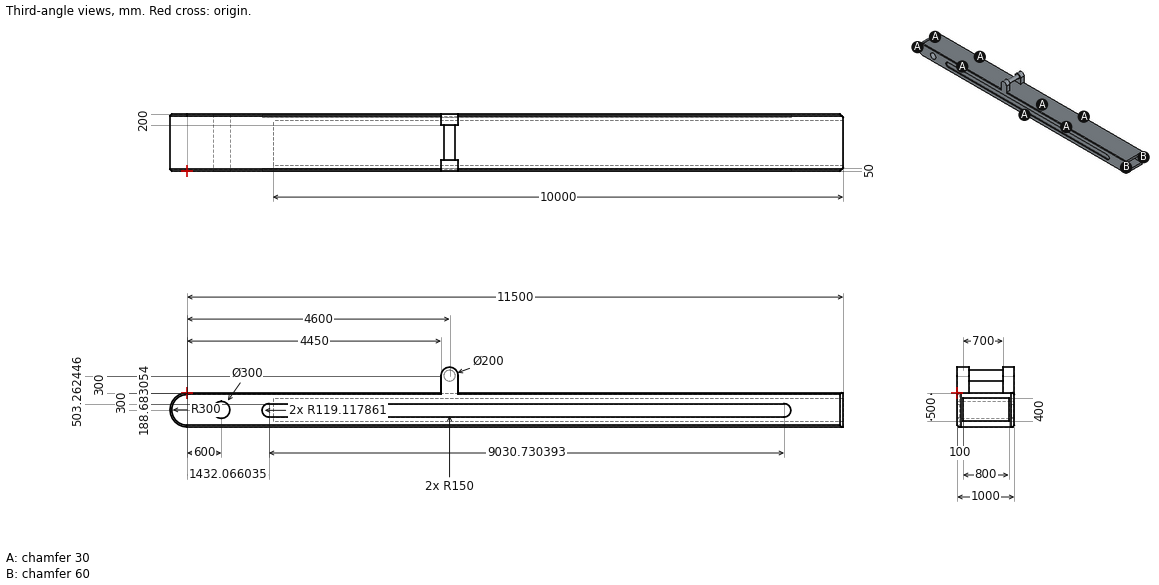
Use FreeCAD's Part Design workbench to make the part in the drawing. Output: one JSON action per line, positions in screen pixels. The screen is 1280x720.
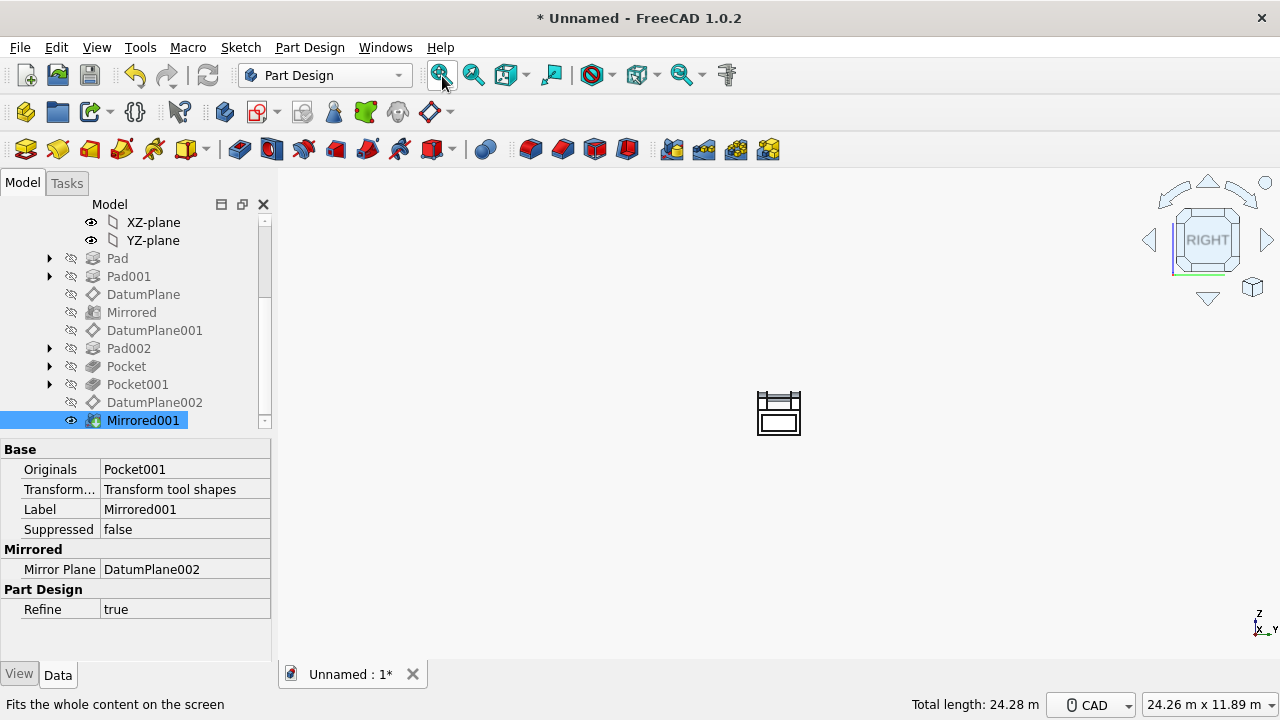
{"action": "key", "text": "5"}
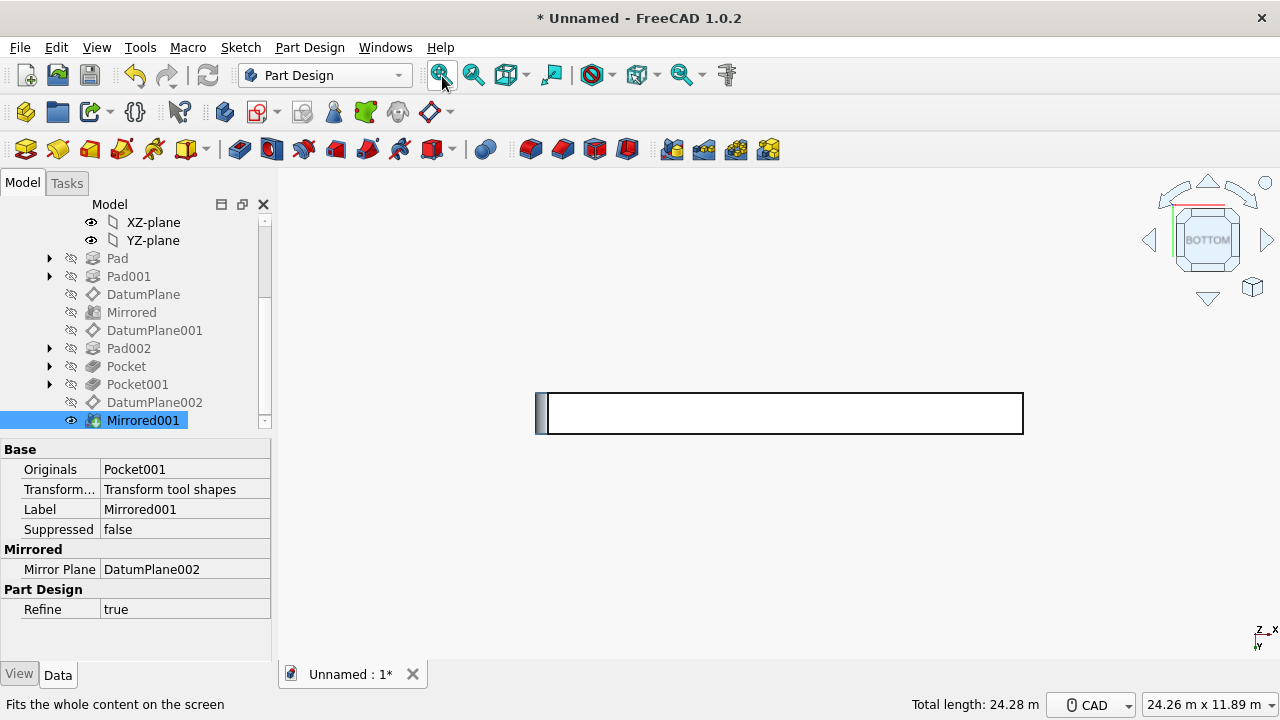
{"action": "left_click", "coordinate": [785, 392], "text": "ctrl"}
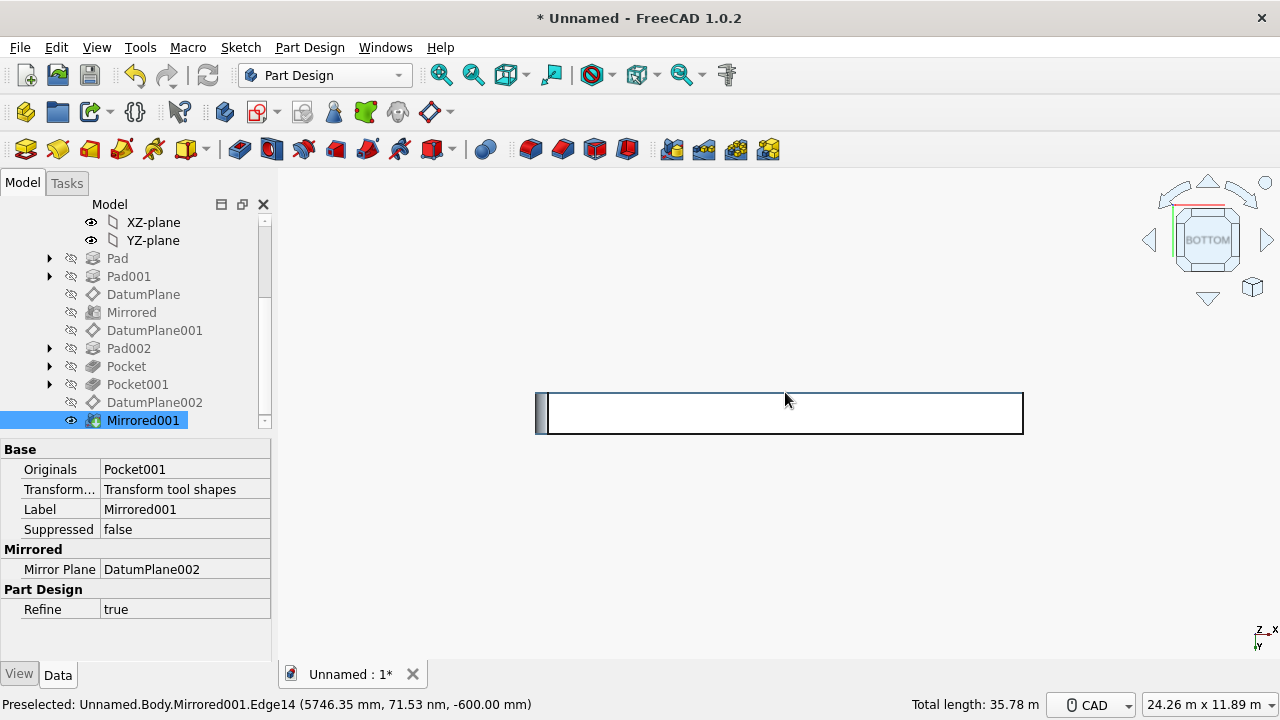
{"action": "key", "text": "4"}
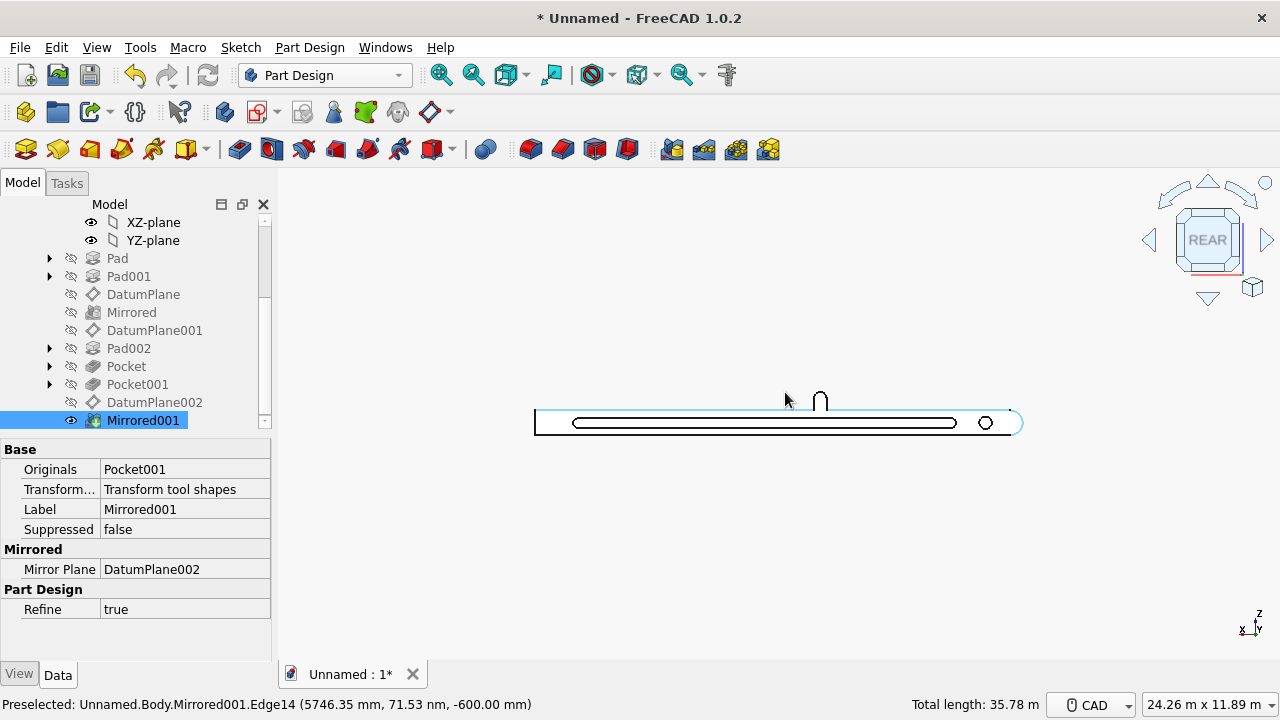
{"action": "left_click", "coordinate": [773, 434], "text": "ctrl"}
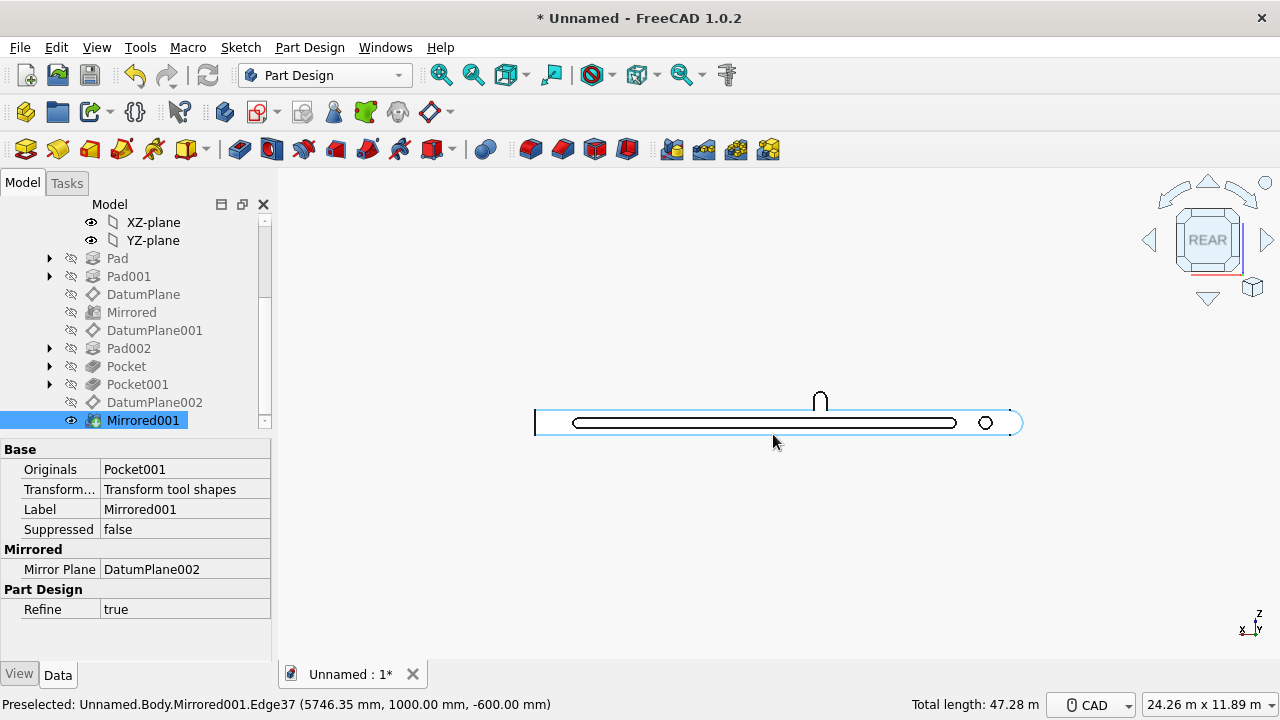
{"action": "left_click", "coordinate": [564, 150]}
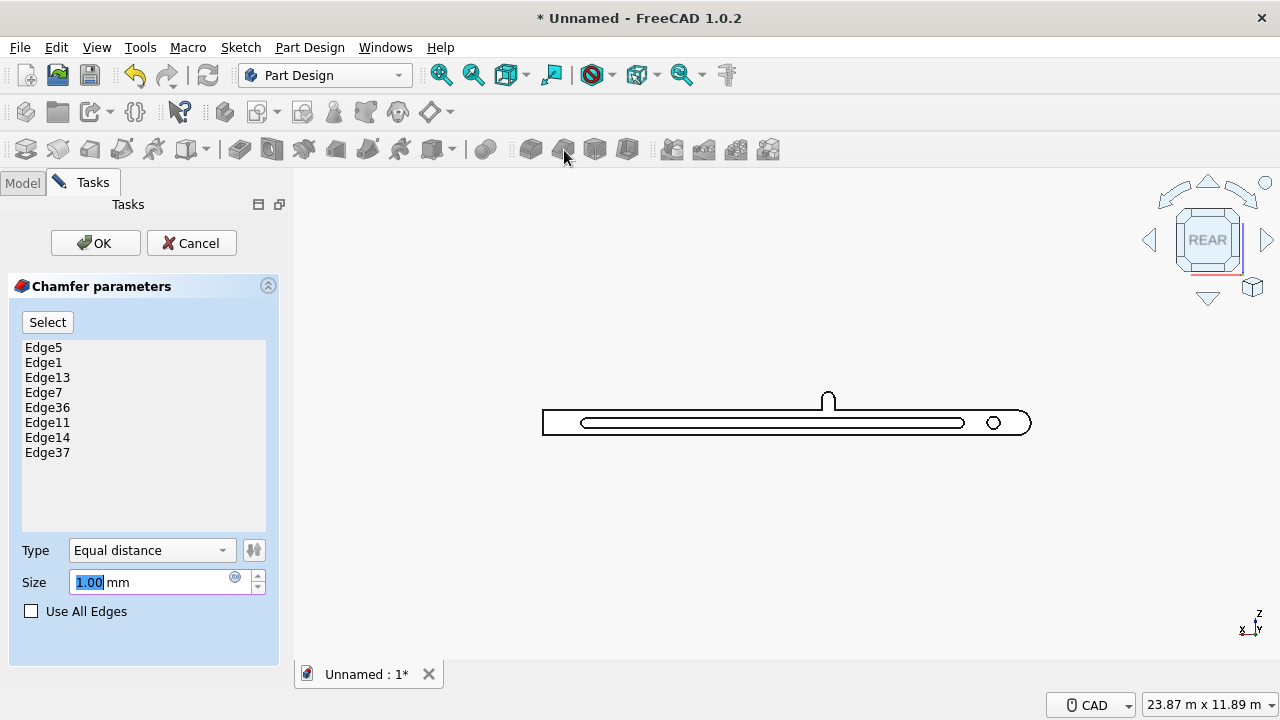
{"action": "type", "text": "30"}
{"action": "key", "text": "Tab"}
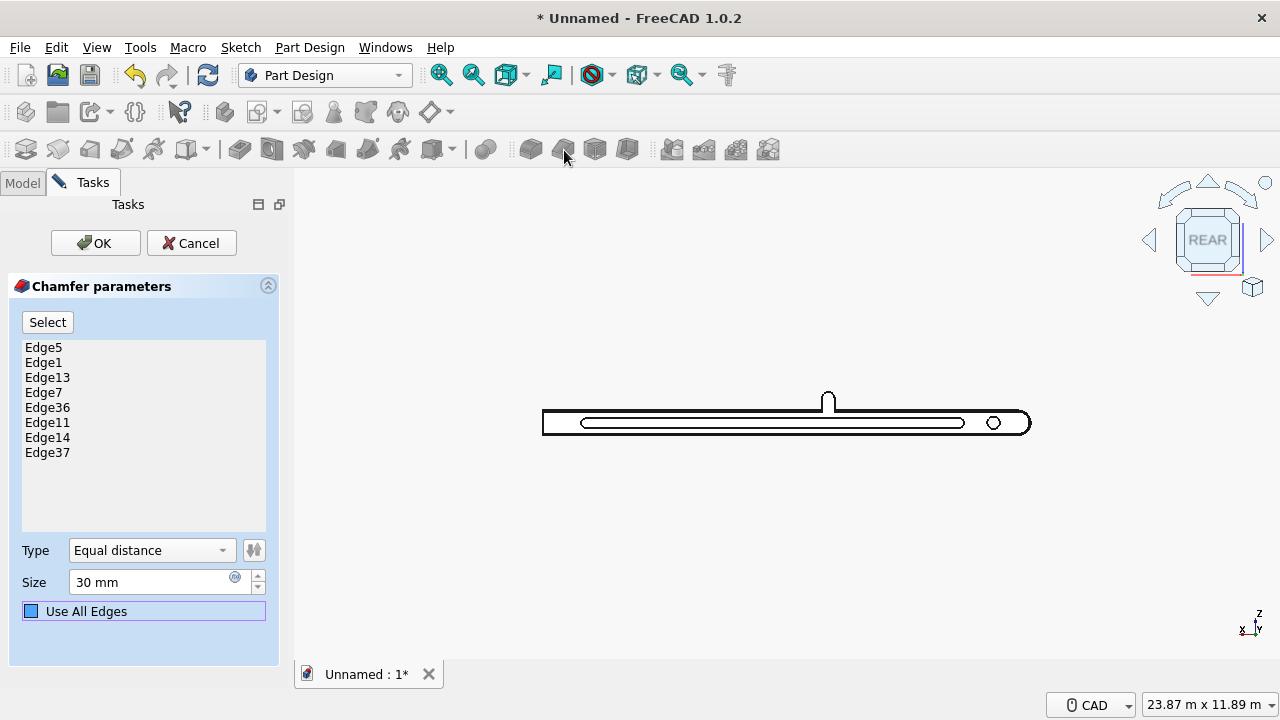
{"action": "left_click", "coordinate": [96, 243]}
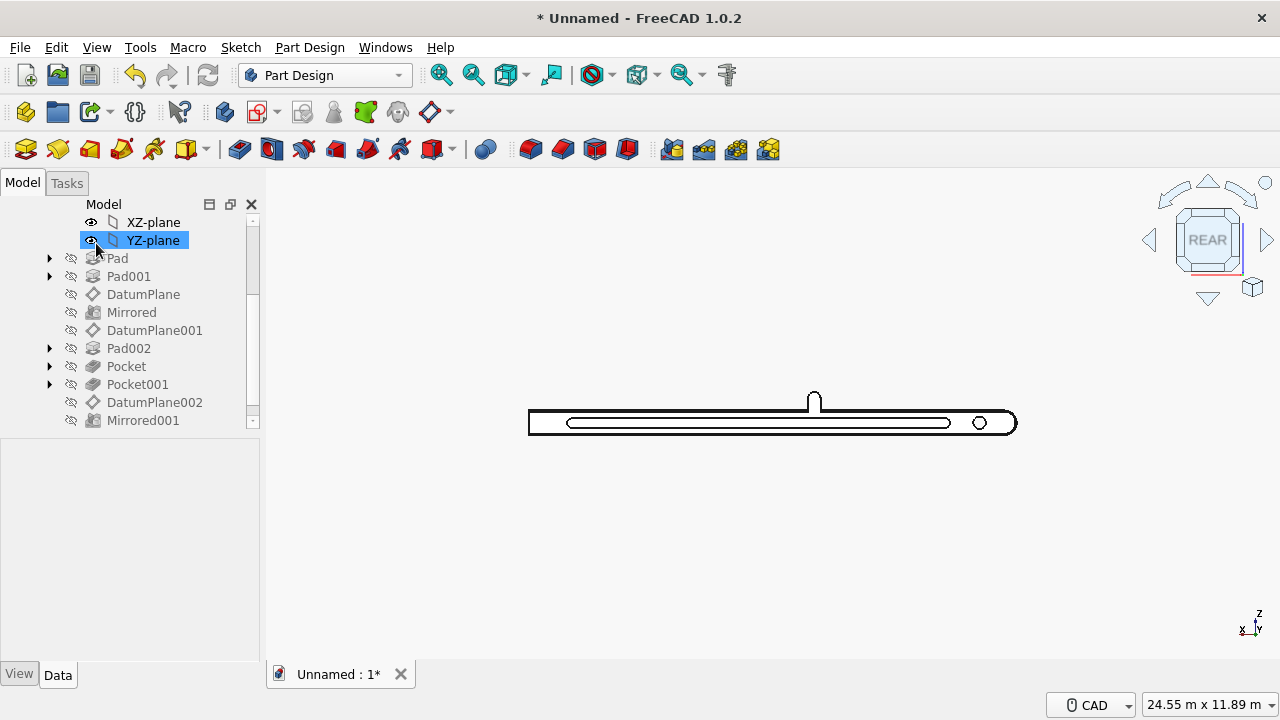
{"action": "left_click", "coordinate": [529, 422]}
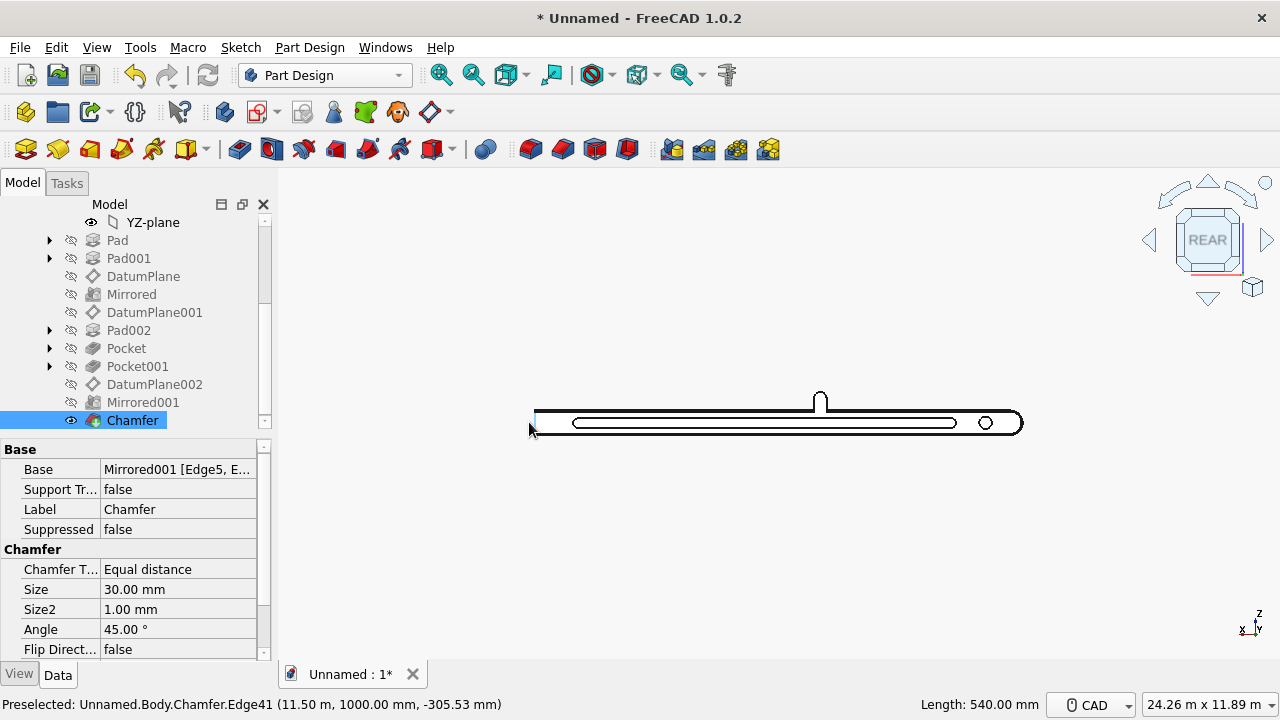
{"action": "key", "text": "0"}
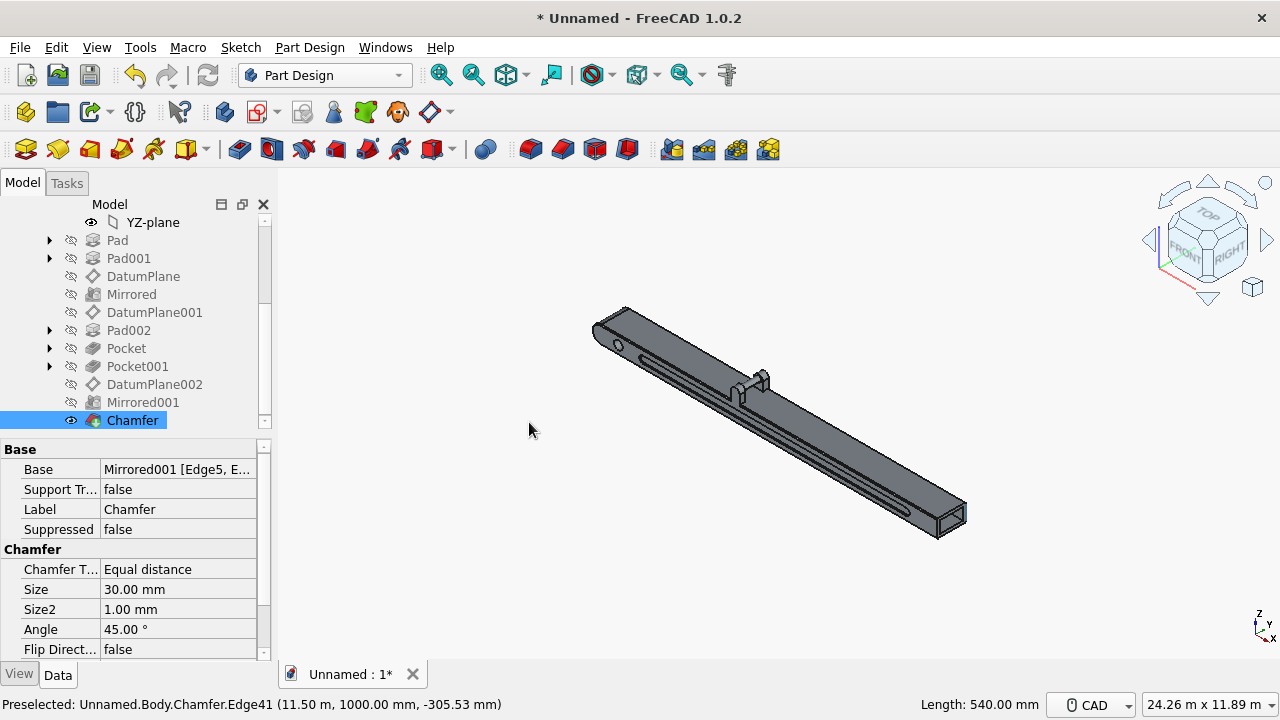
{"action": "left_click", "coordinate": [937, 528], "text": "ctrl"}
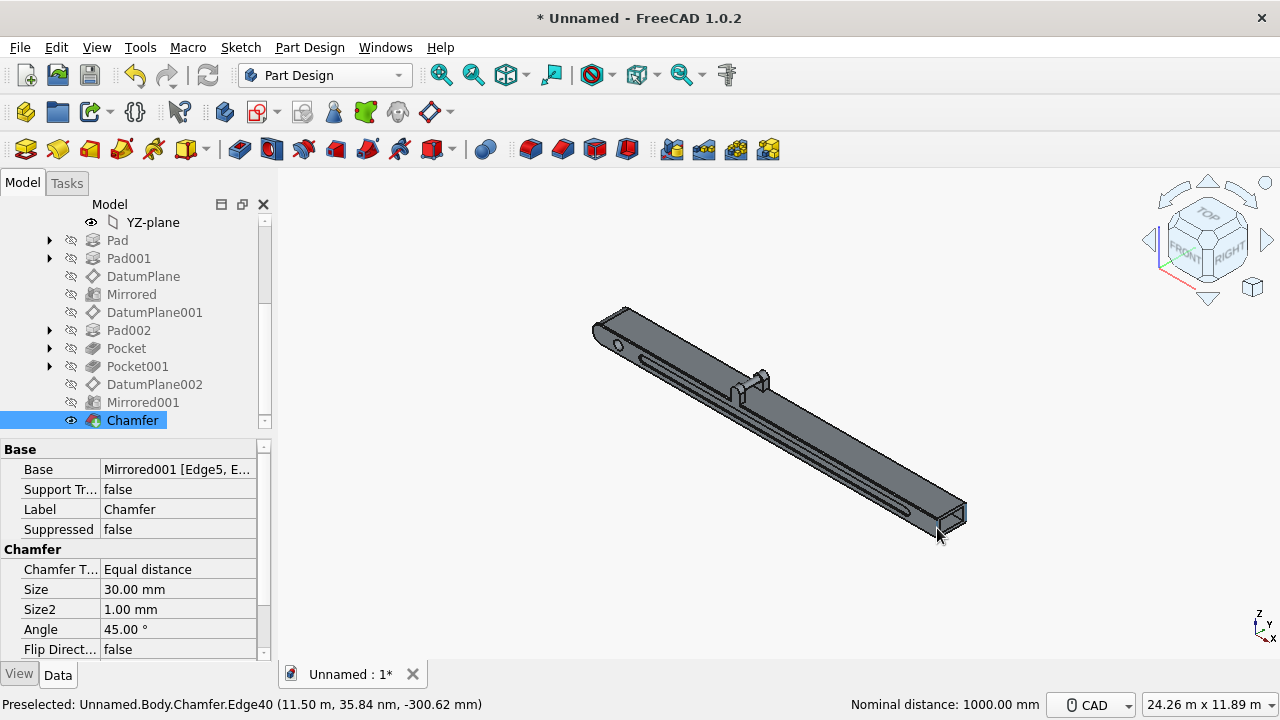
{"action": "left_click", "coordinate": [564, 150]}